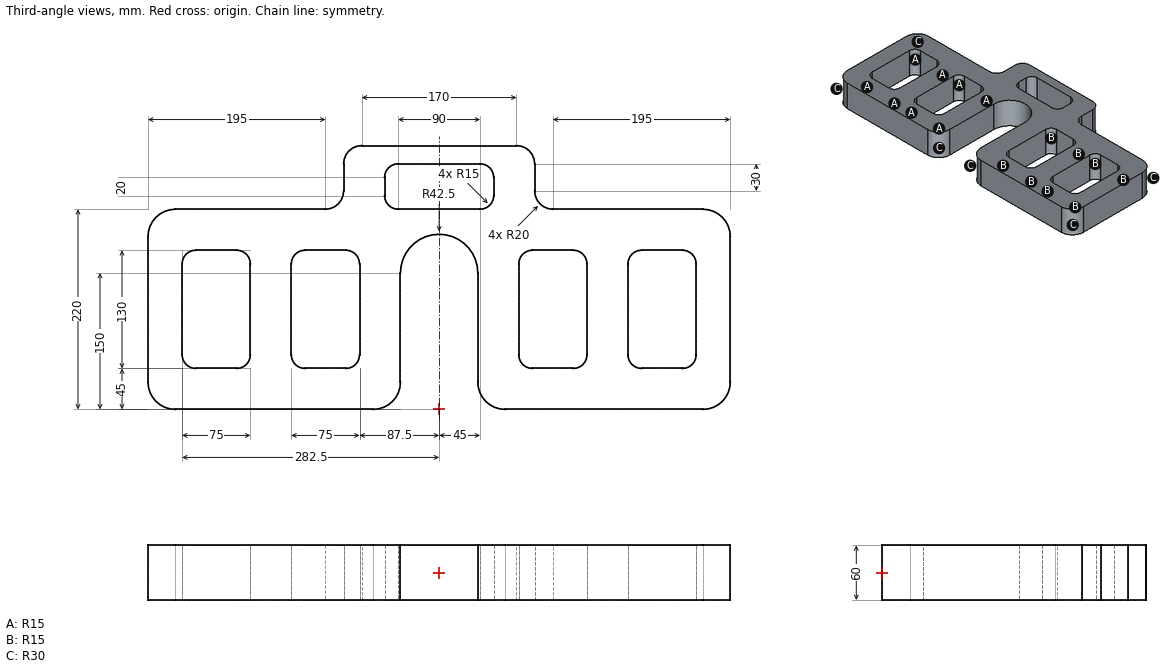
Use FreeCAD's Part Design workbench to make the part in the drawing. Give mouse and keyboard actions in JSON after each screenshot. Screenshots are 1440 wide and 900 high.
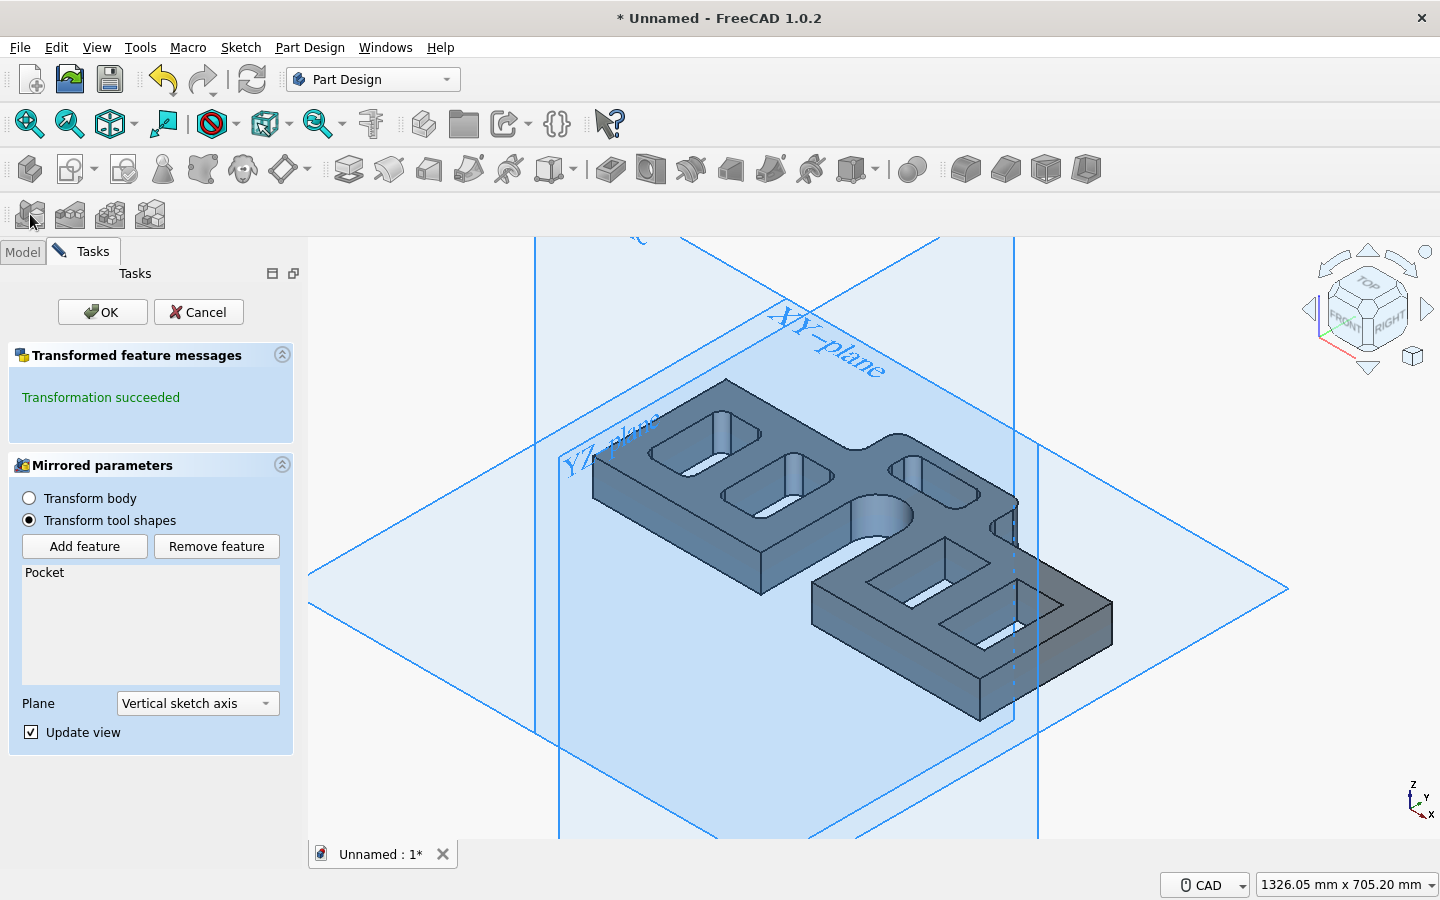
{"action": "left_click", "coordinate": [198, 704]}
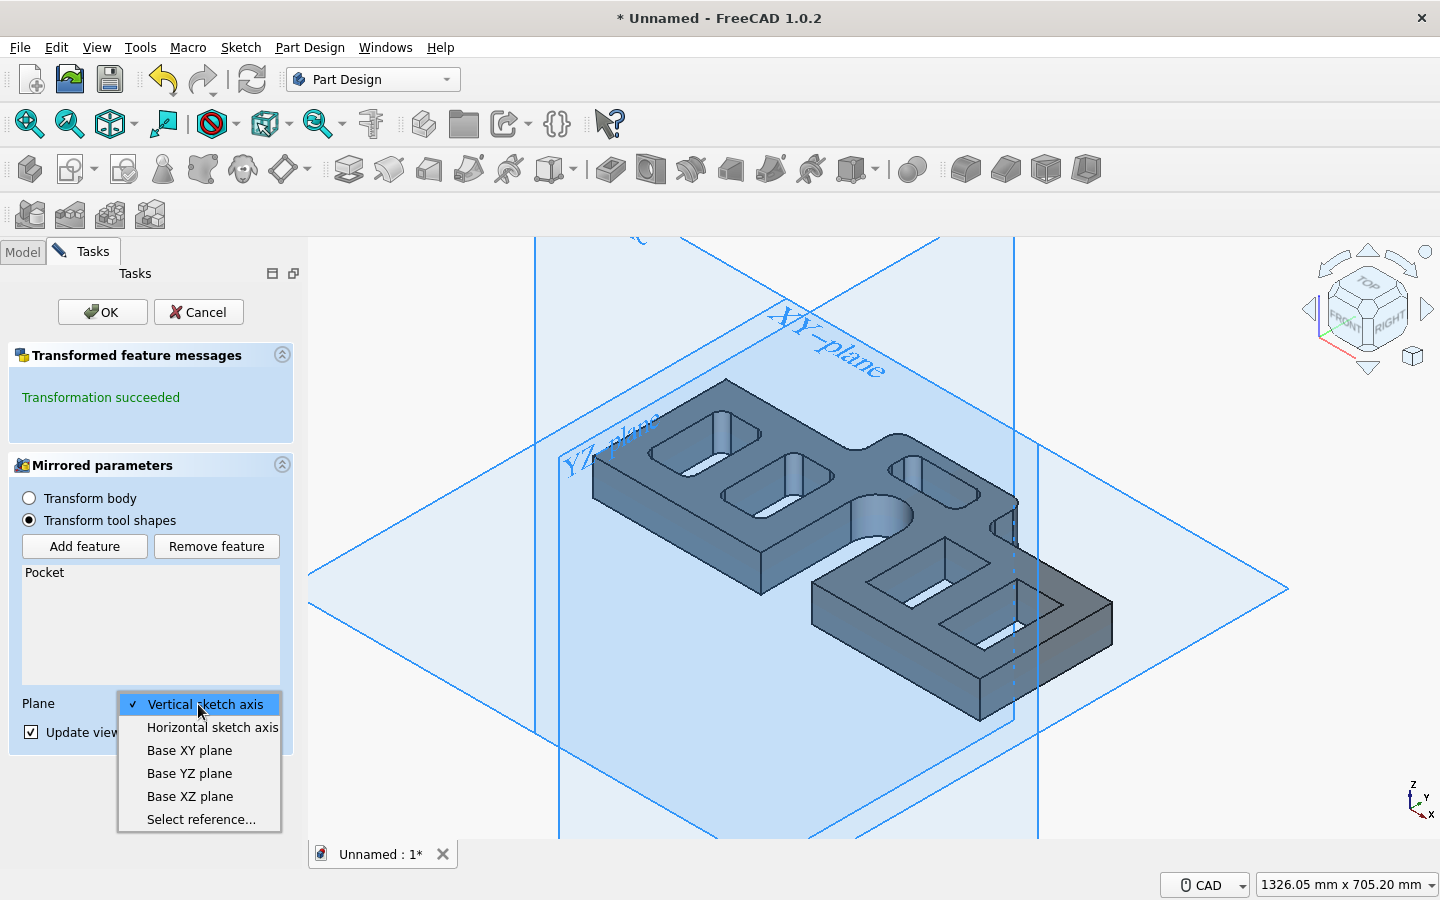
{"action": "left_click", "coordinate": [198, 774]}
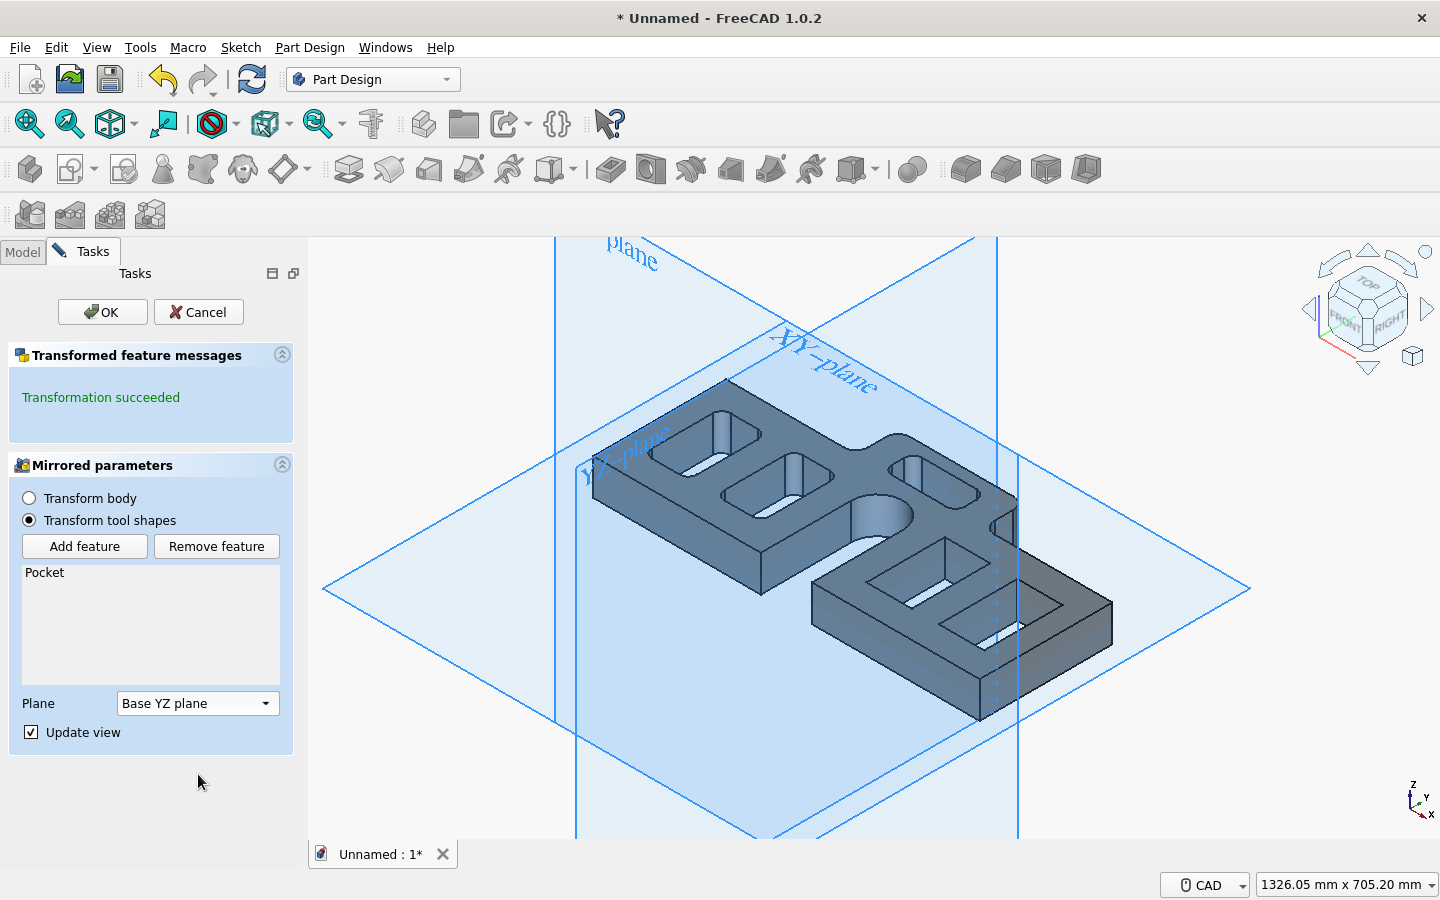
{"action": "left_click", "coordinate": [103, 312]}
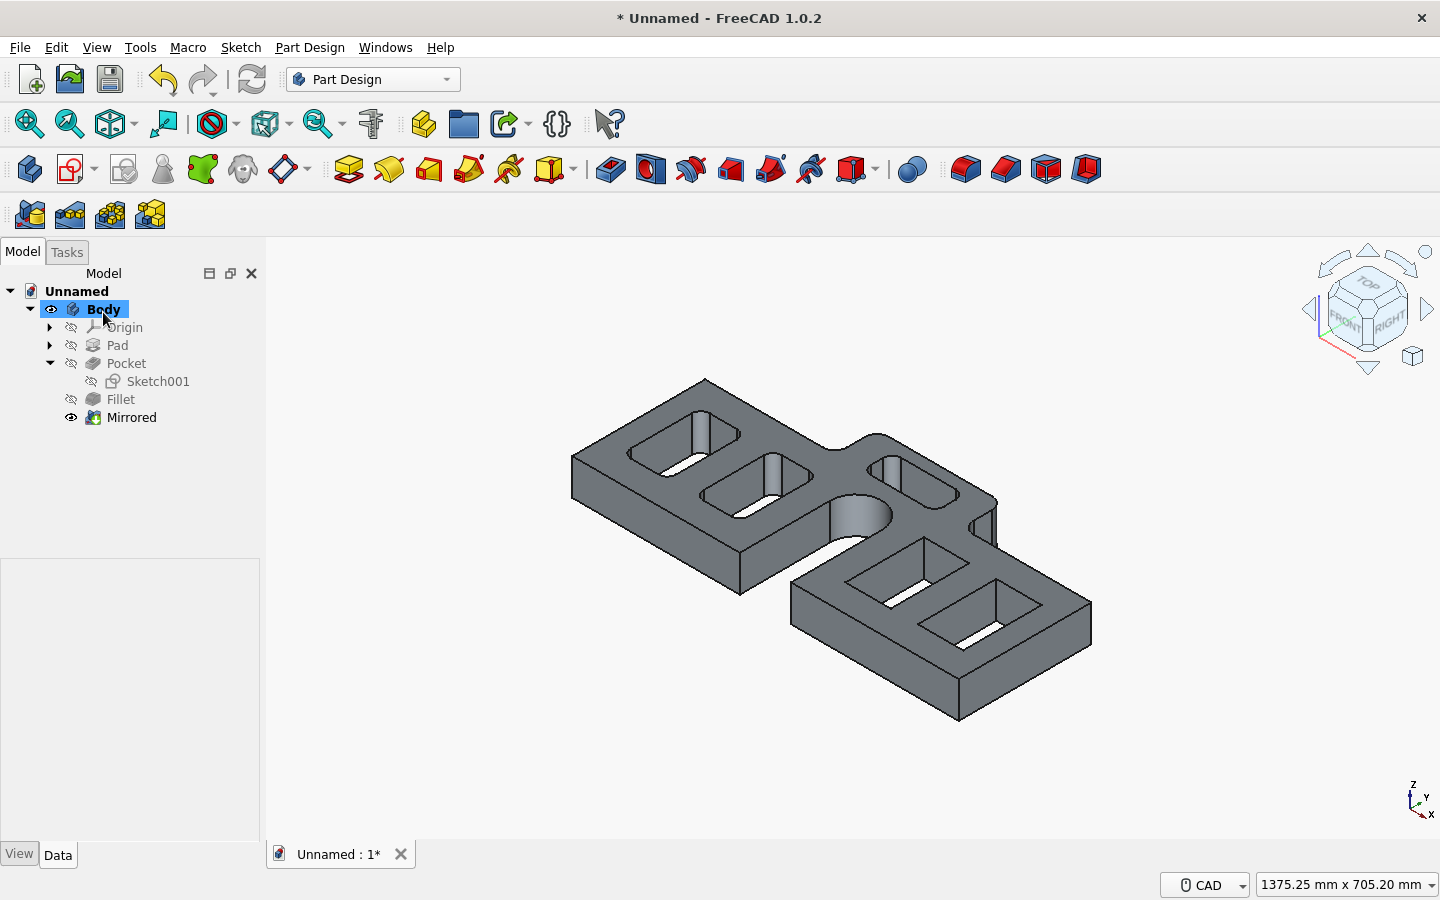
{"action": "key", "text": "2"}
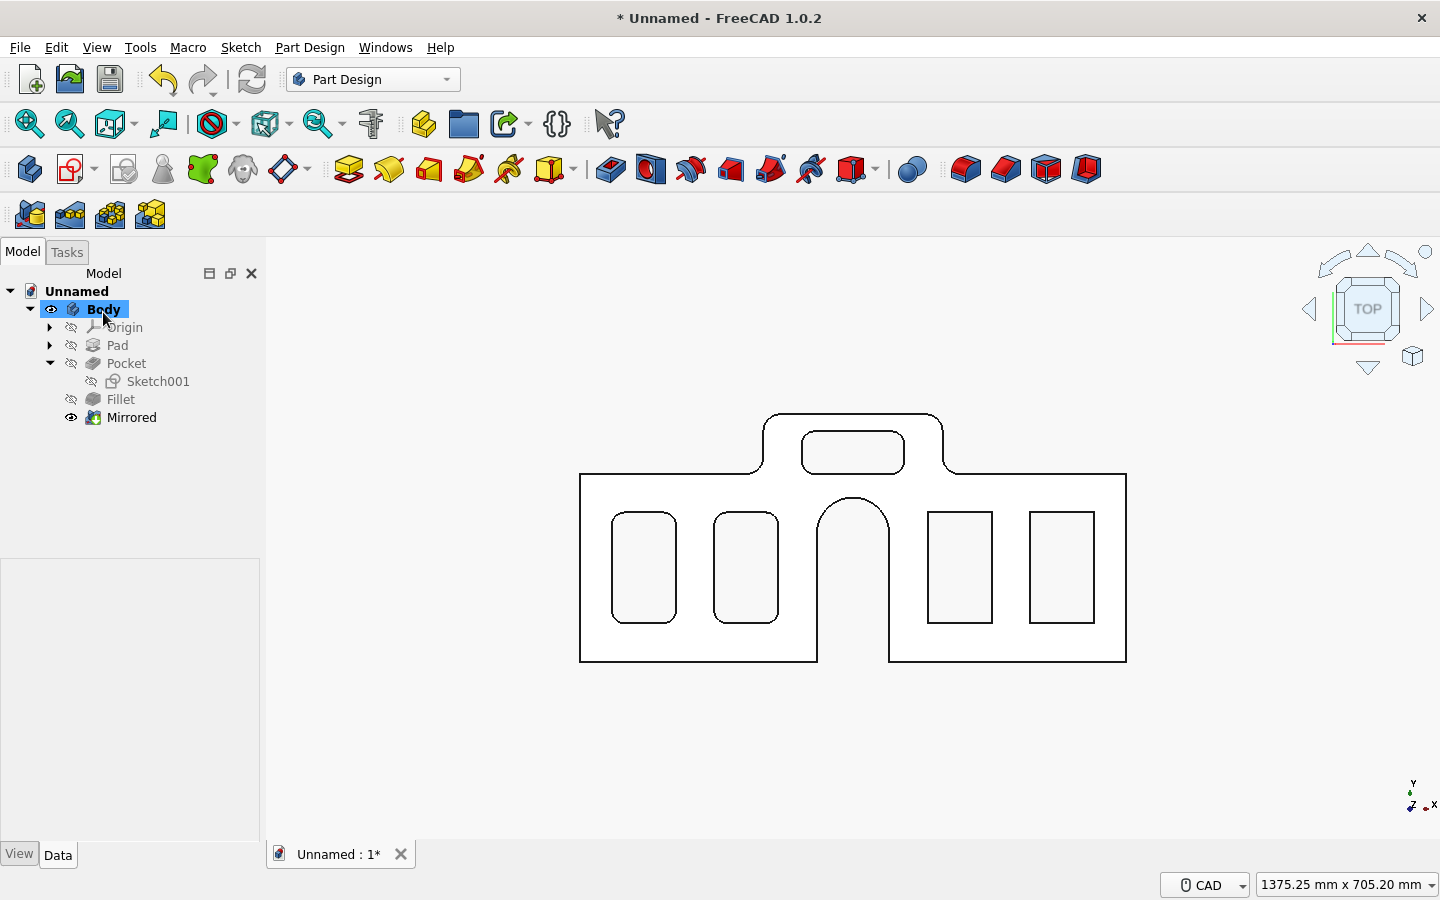
{"action": "key", "text": "0"}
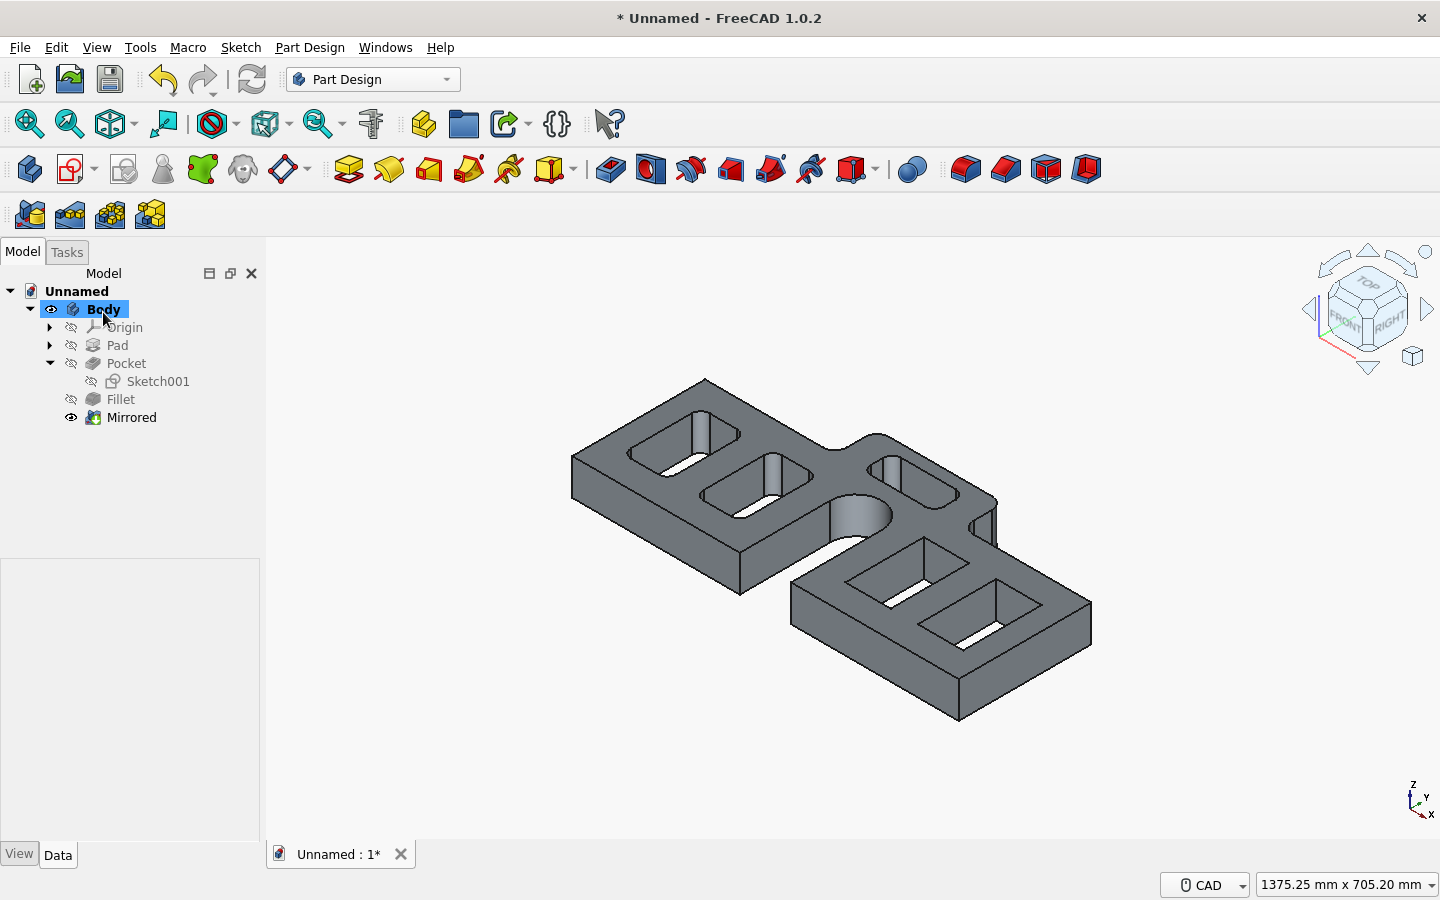
{"action": "key", "text": "1"}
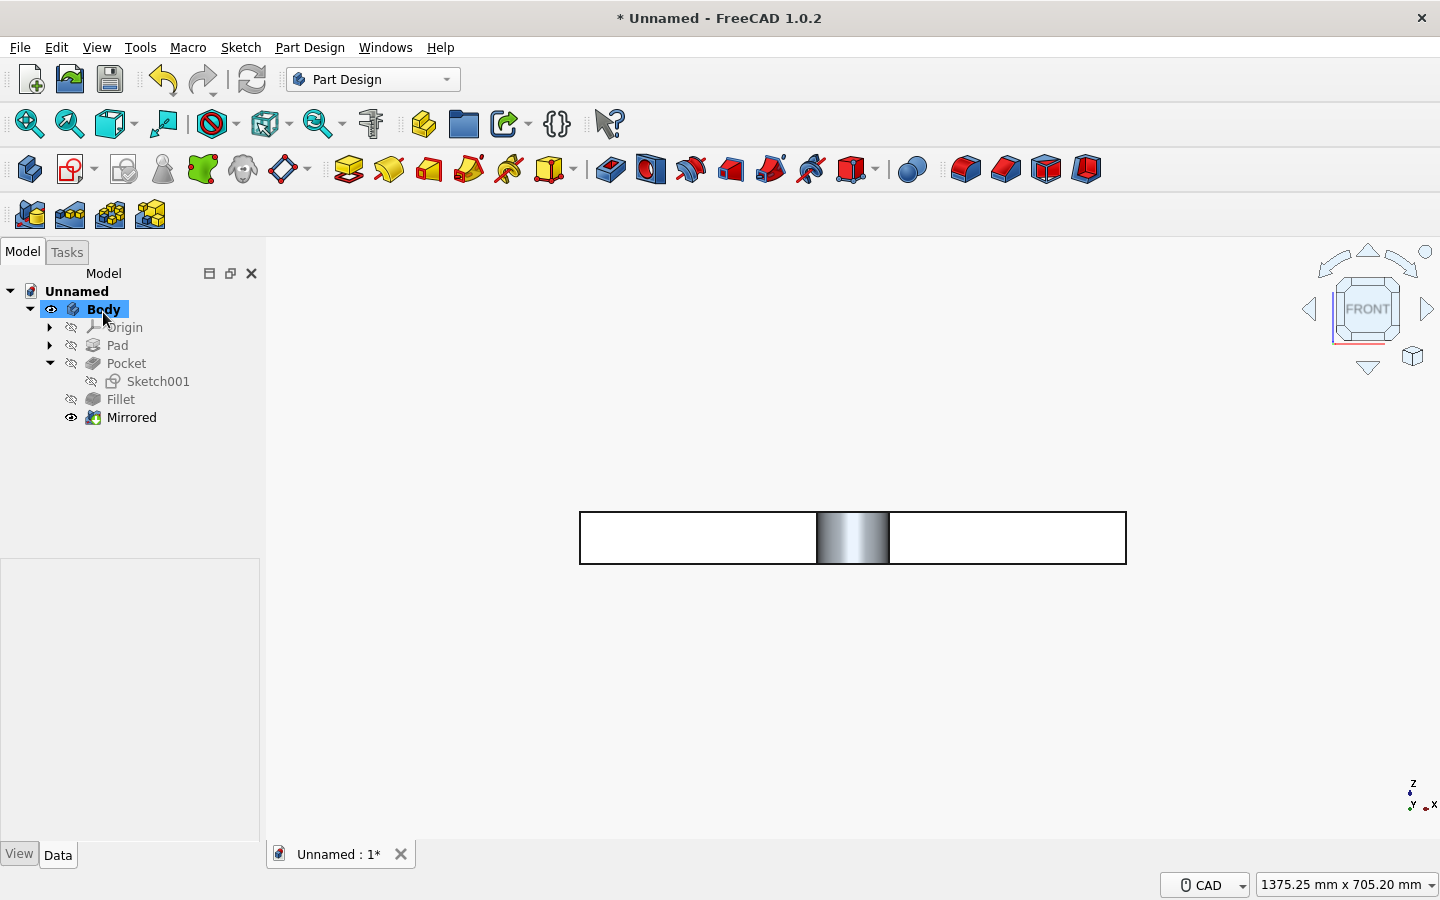
{"action": "key", "text": "3"}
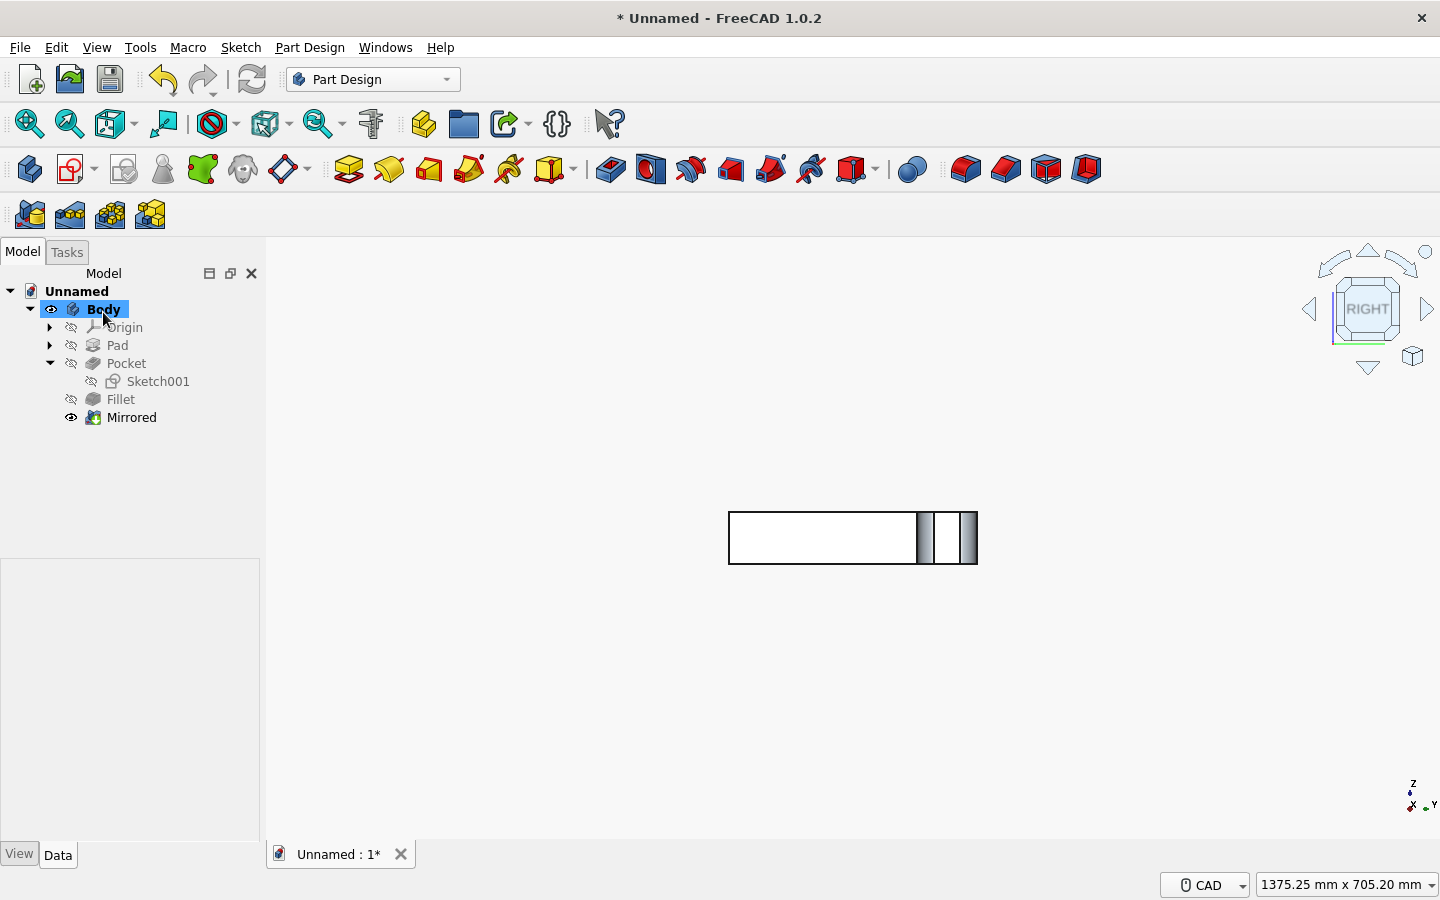
{"action": "key", "text": "v f"}